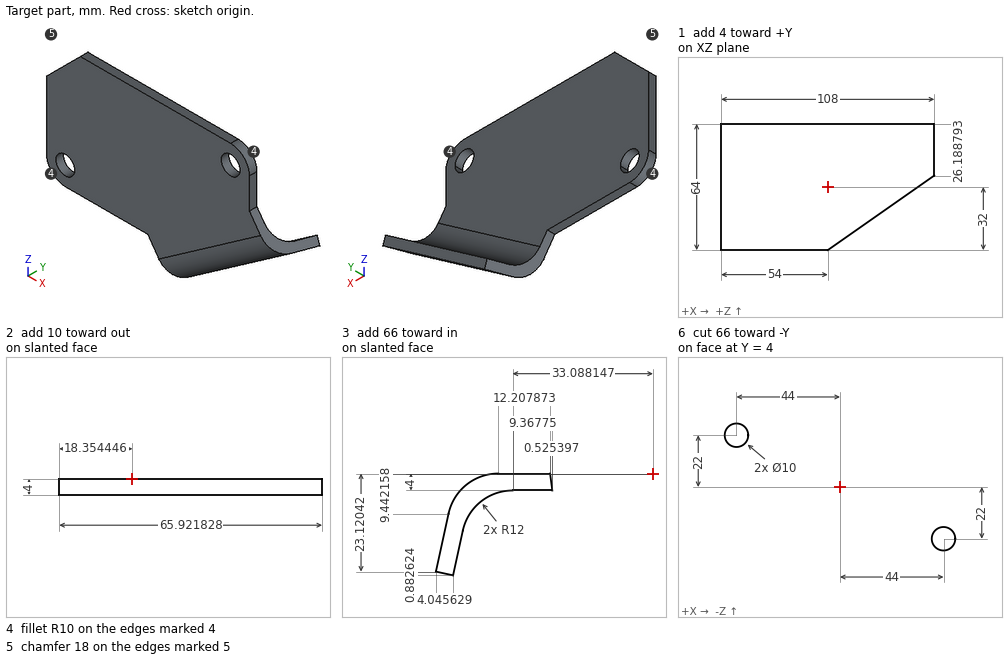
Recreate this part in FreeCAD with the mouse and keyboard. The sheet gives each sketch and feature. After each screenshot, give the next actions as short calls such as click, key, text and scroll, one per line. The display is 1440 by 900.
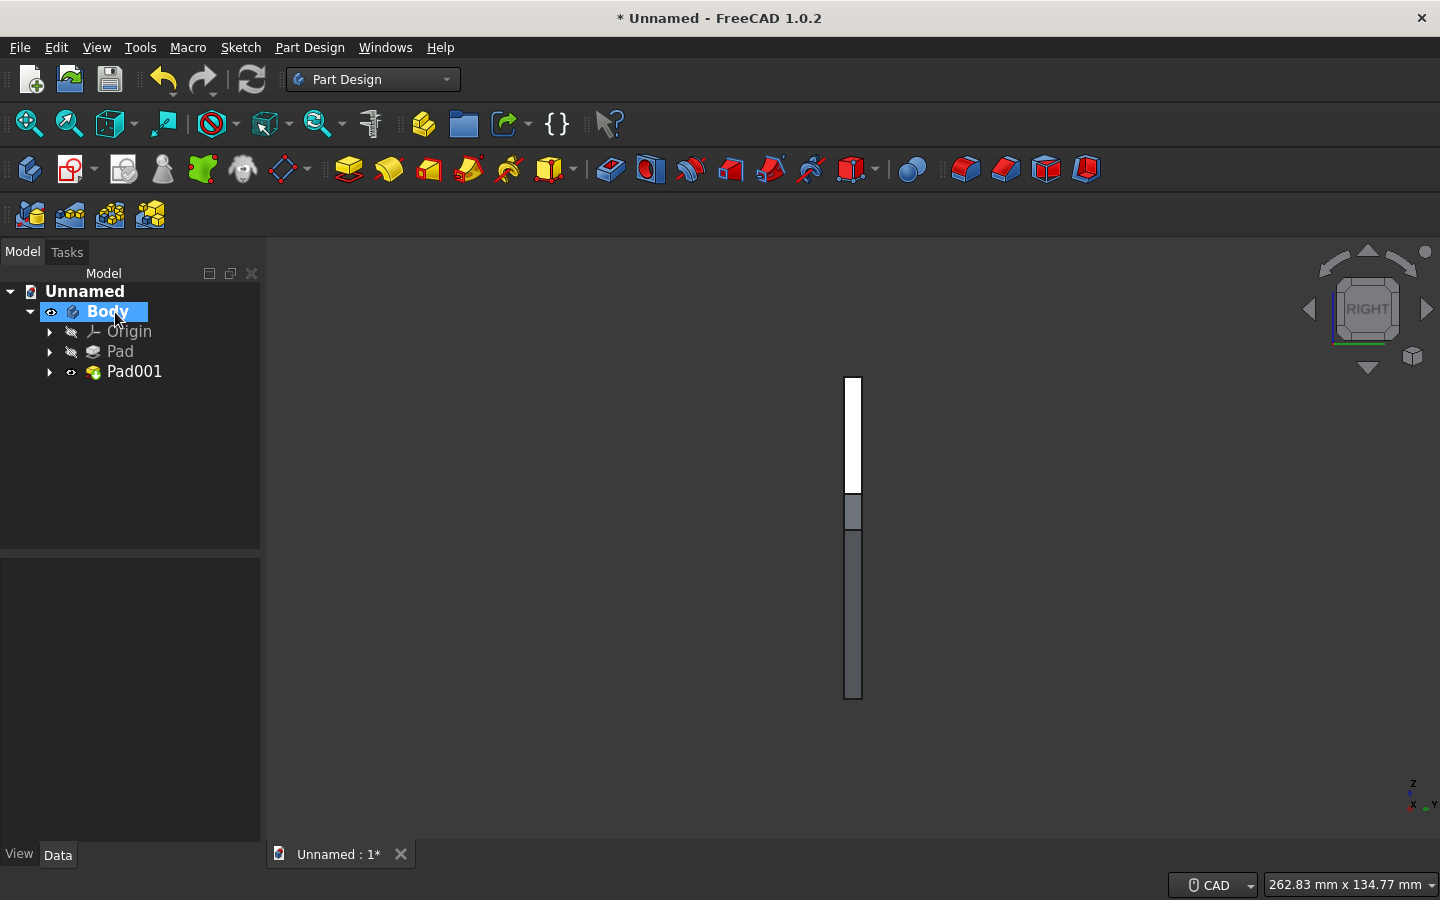
click(853, 516)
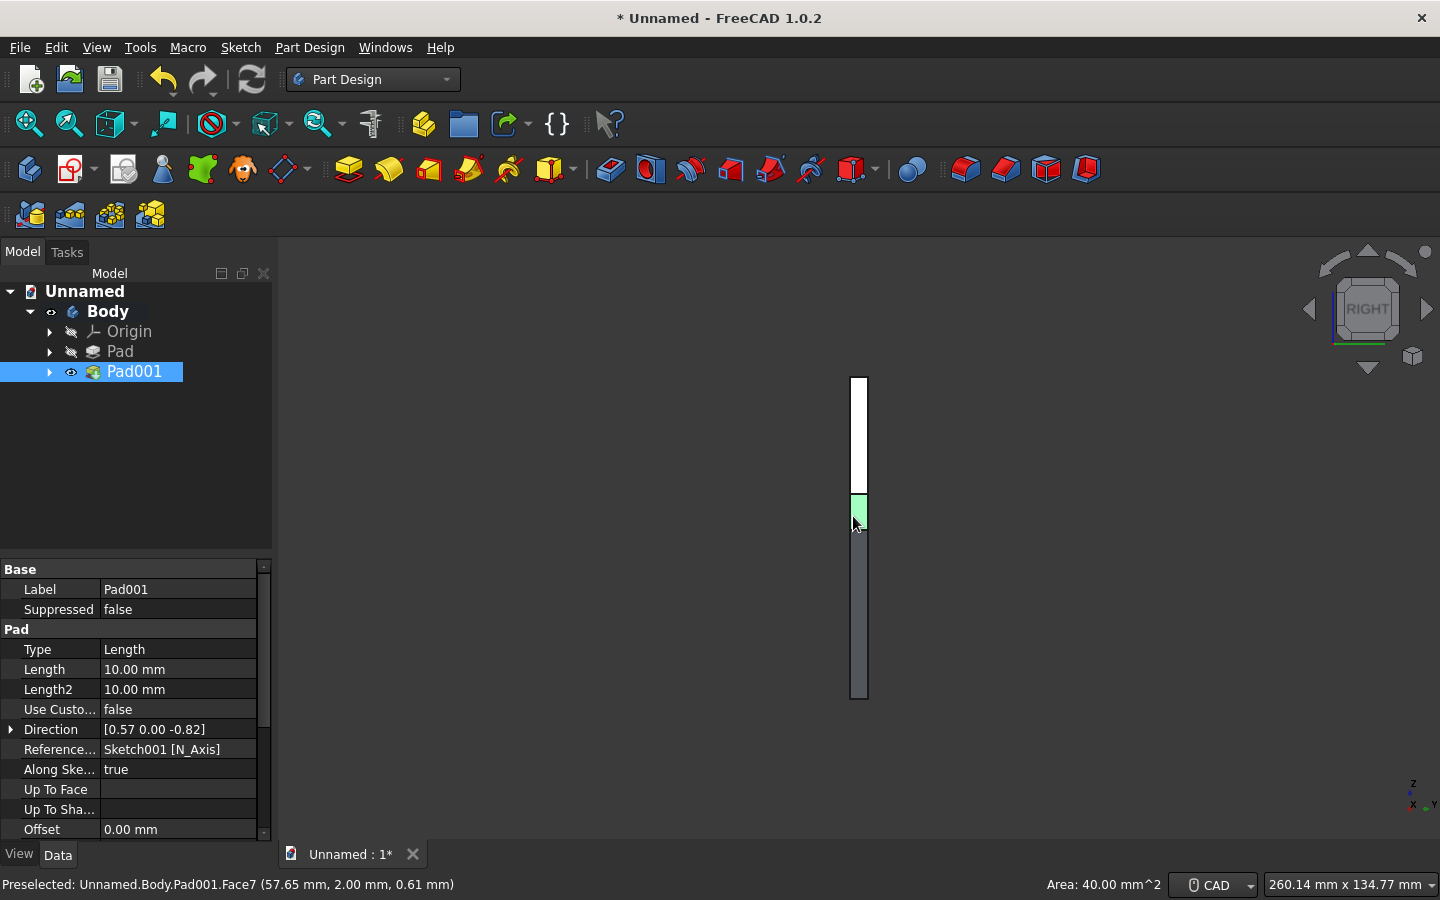
click(70, 170)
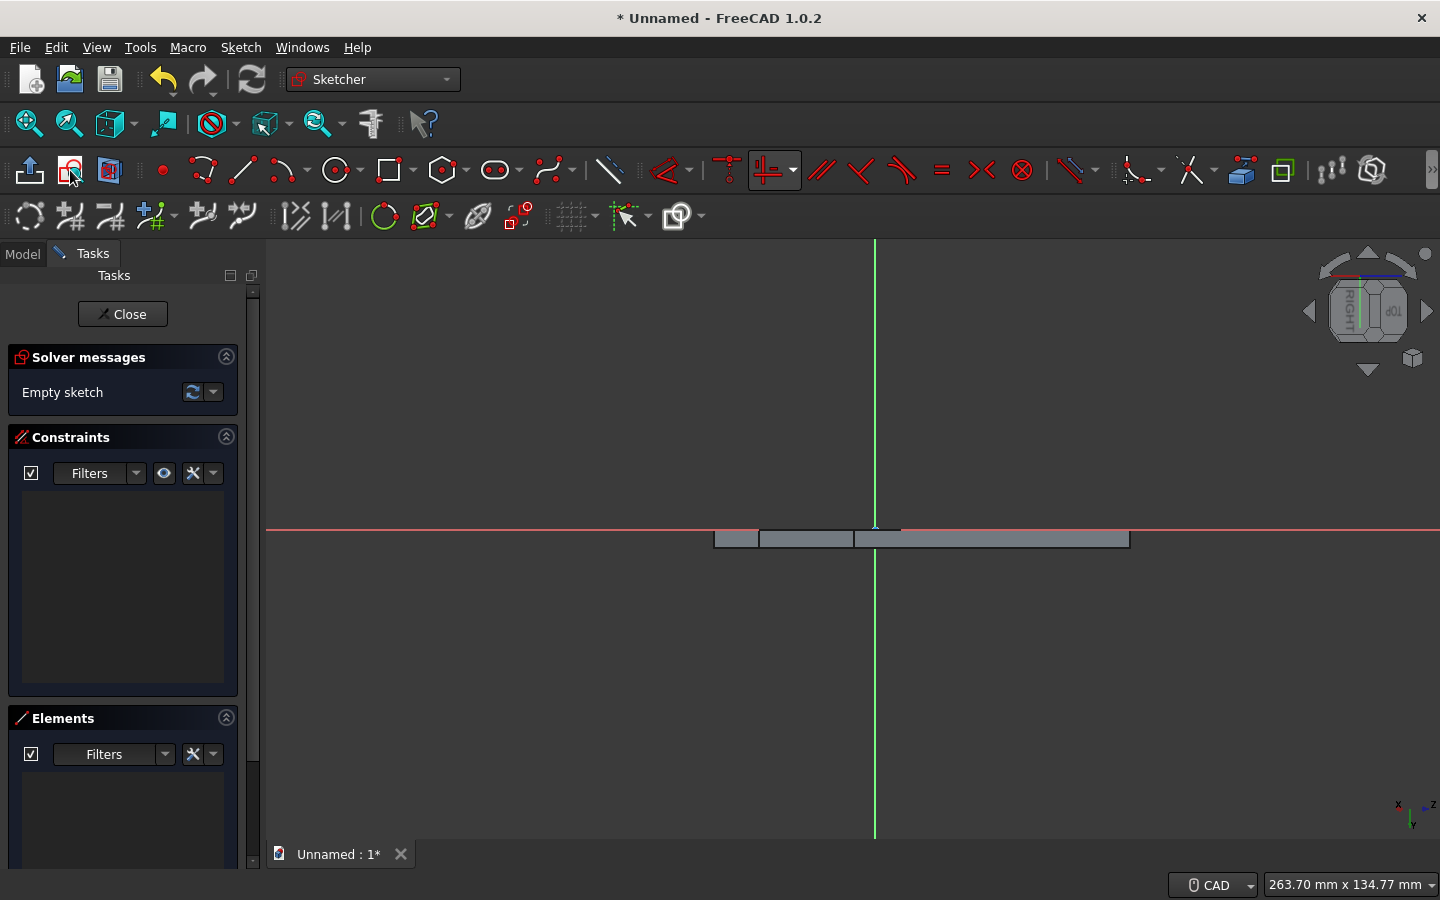
scroll(751, 603, up, 6)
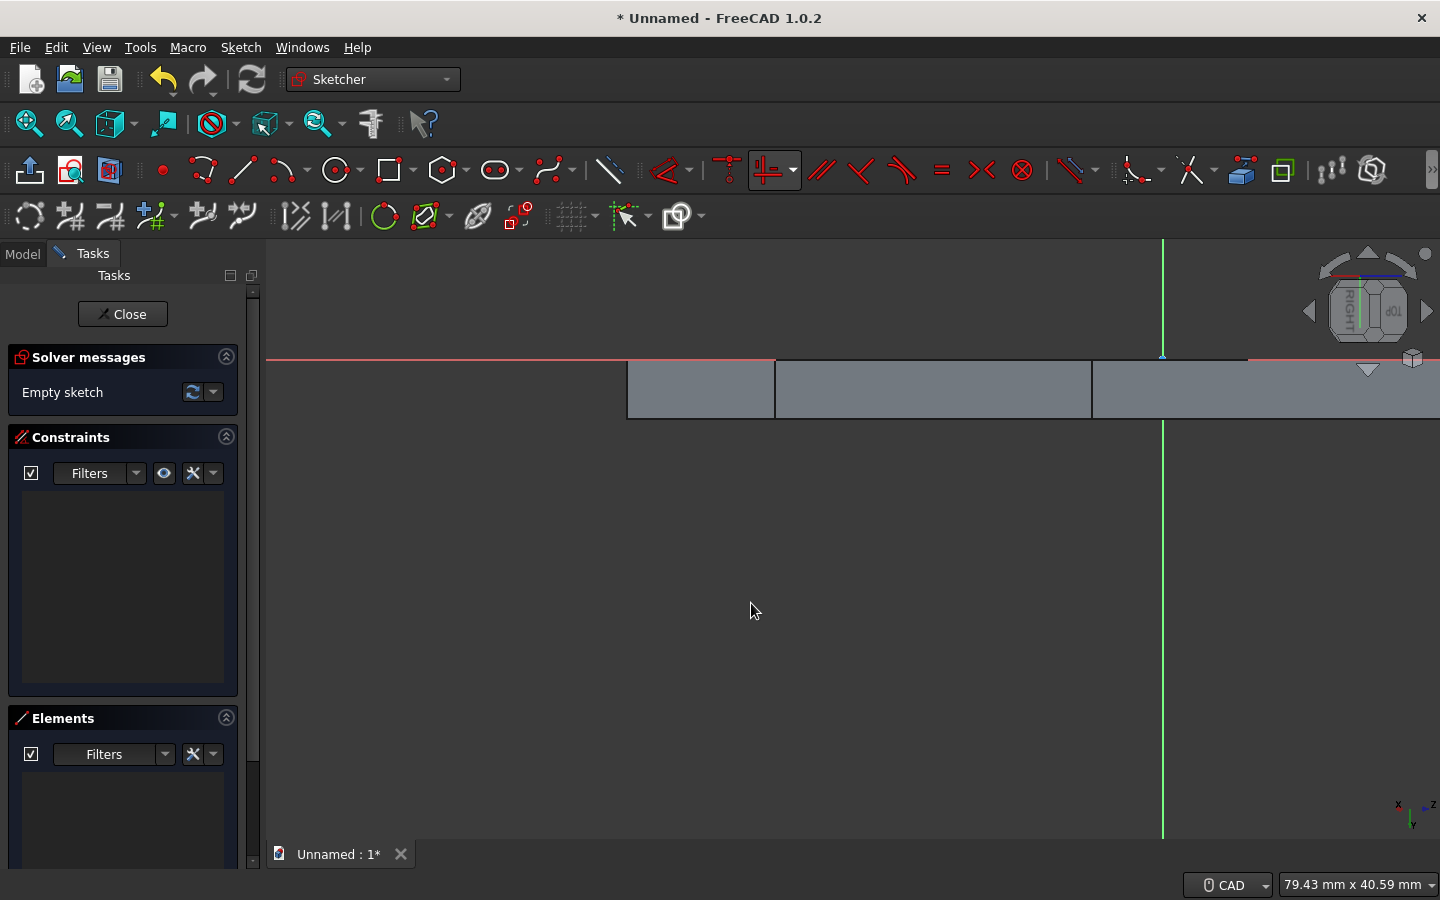
key(g)
key(m)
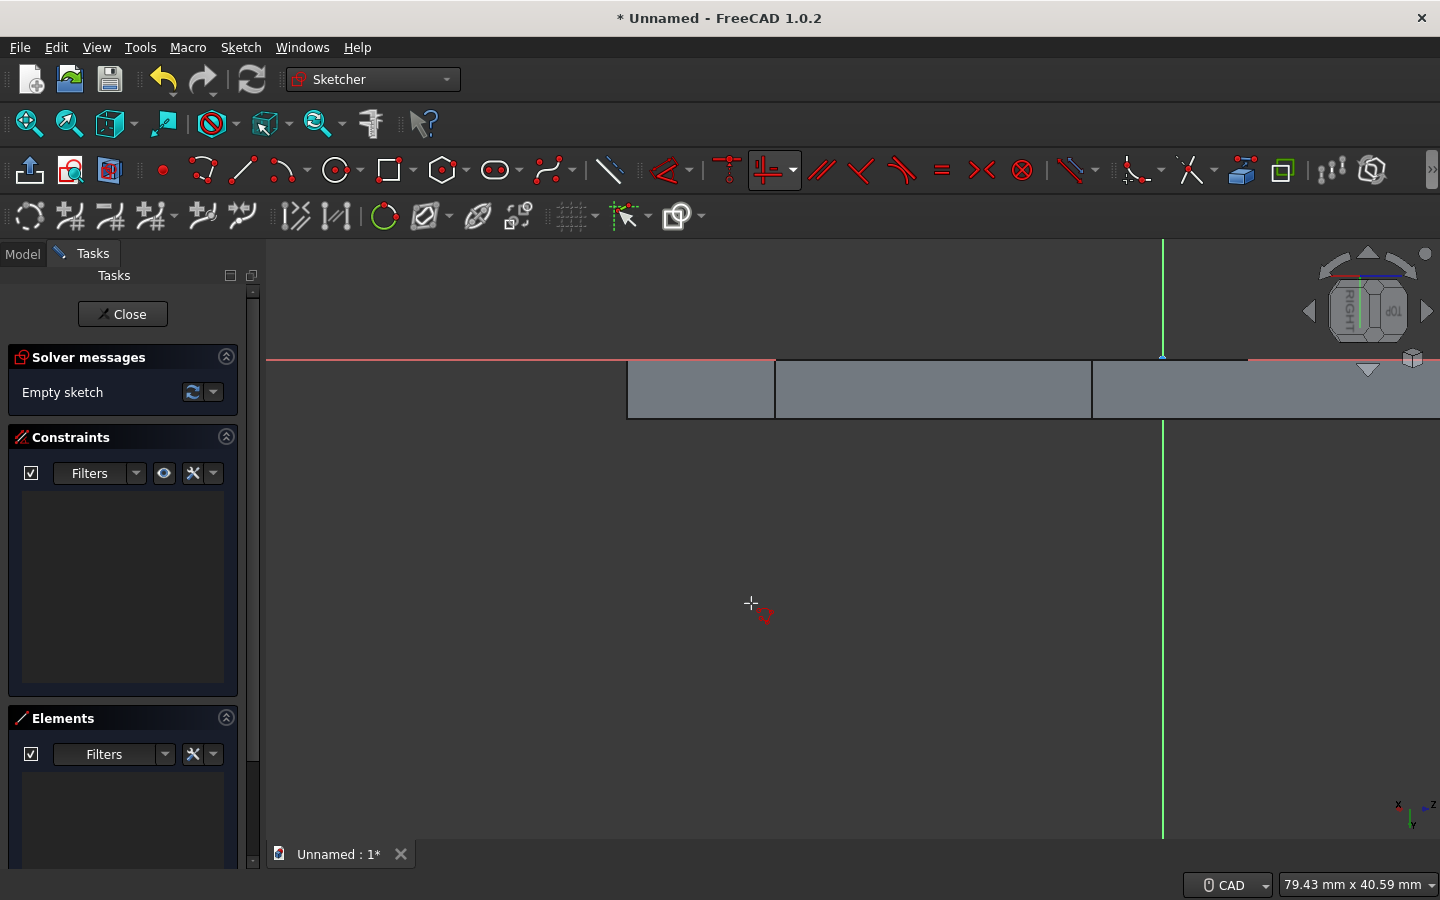
click(674, 419)
click(812, 419)
click(804, 360)
click(624, 369)
right_click(624, 369)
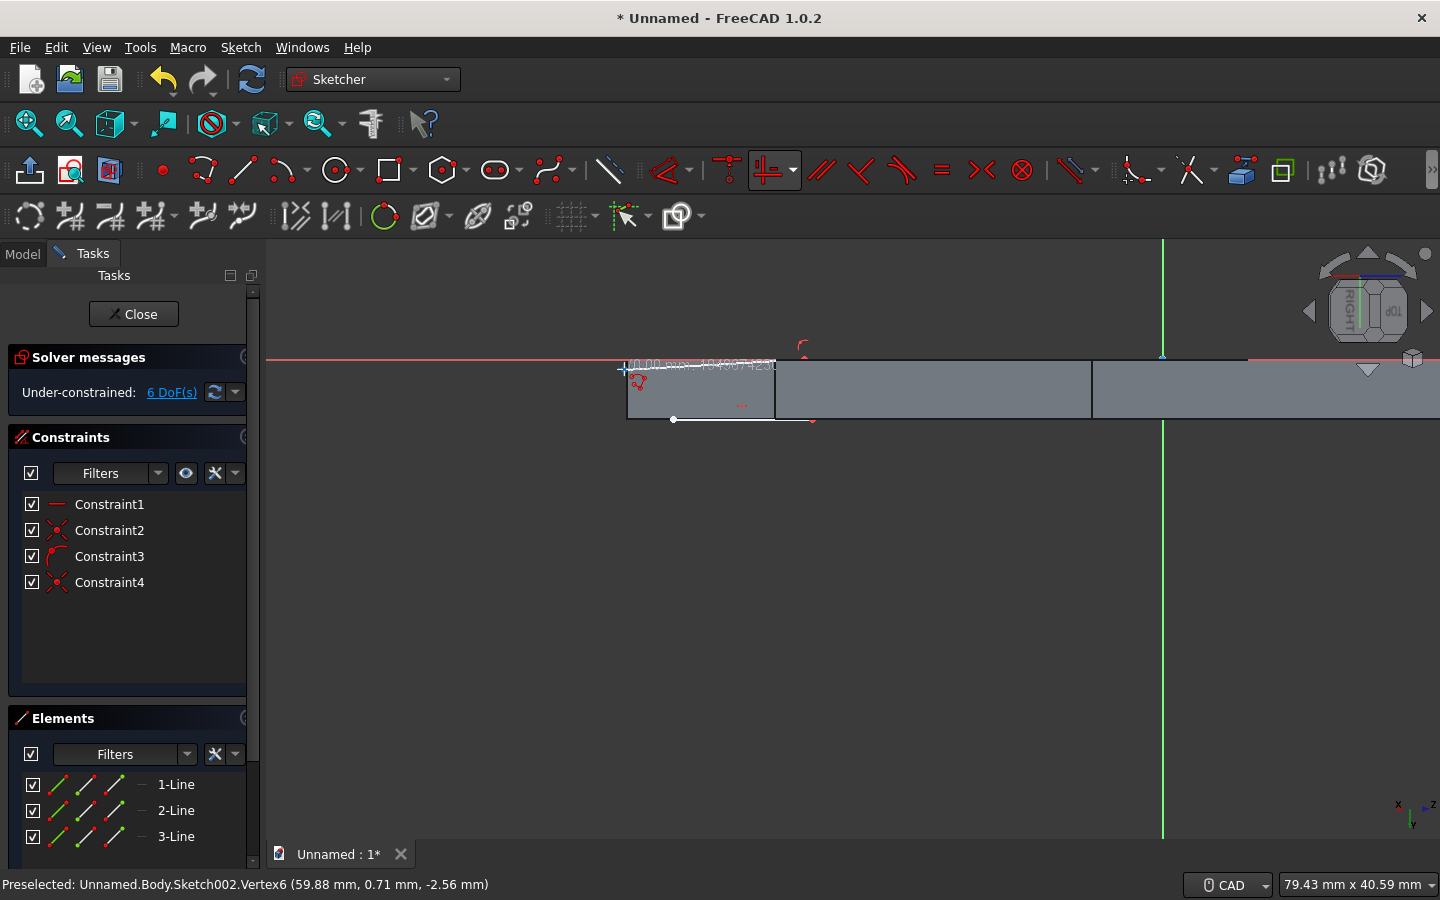
click(450, 499)
click(406, 701)
click(466, 714)
click(500, 558)
right_click(500, 558)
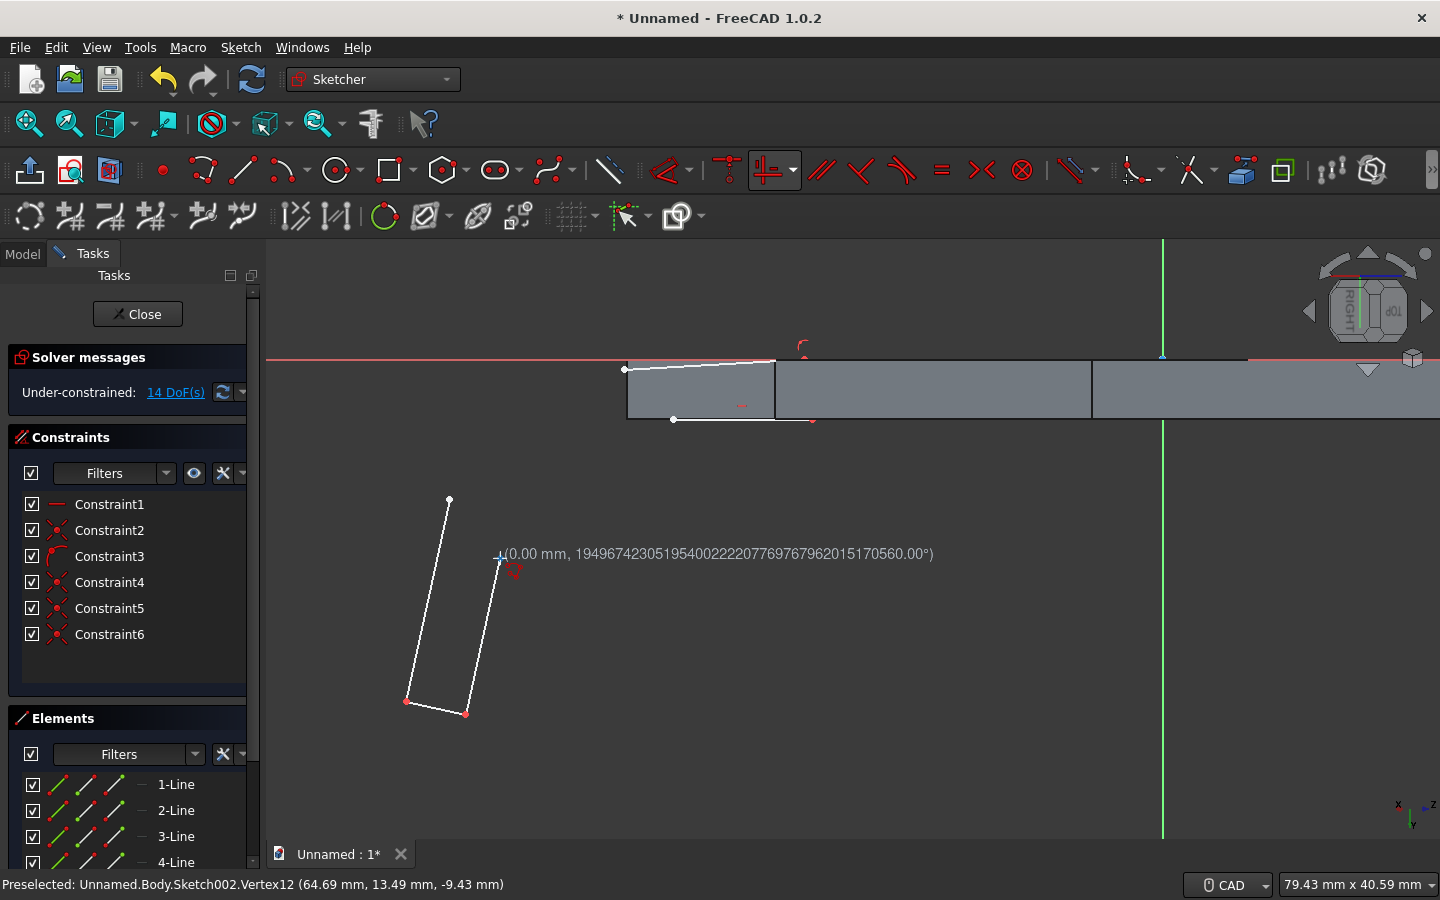
key(g)
key(3)
key(a)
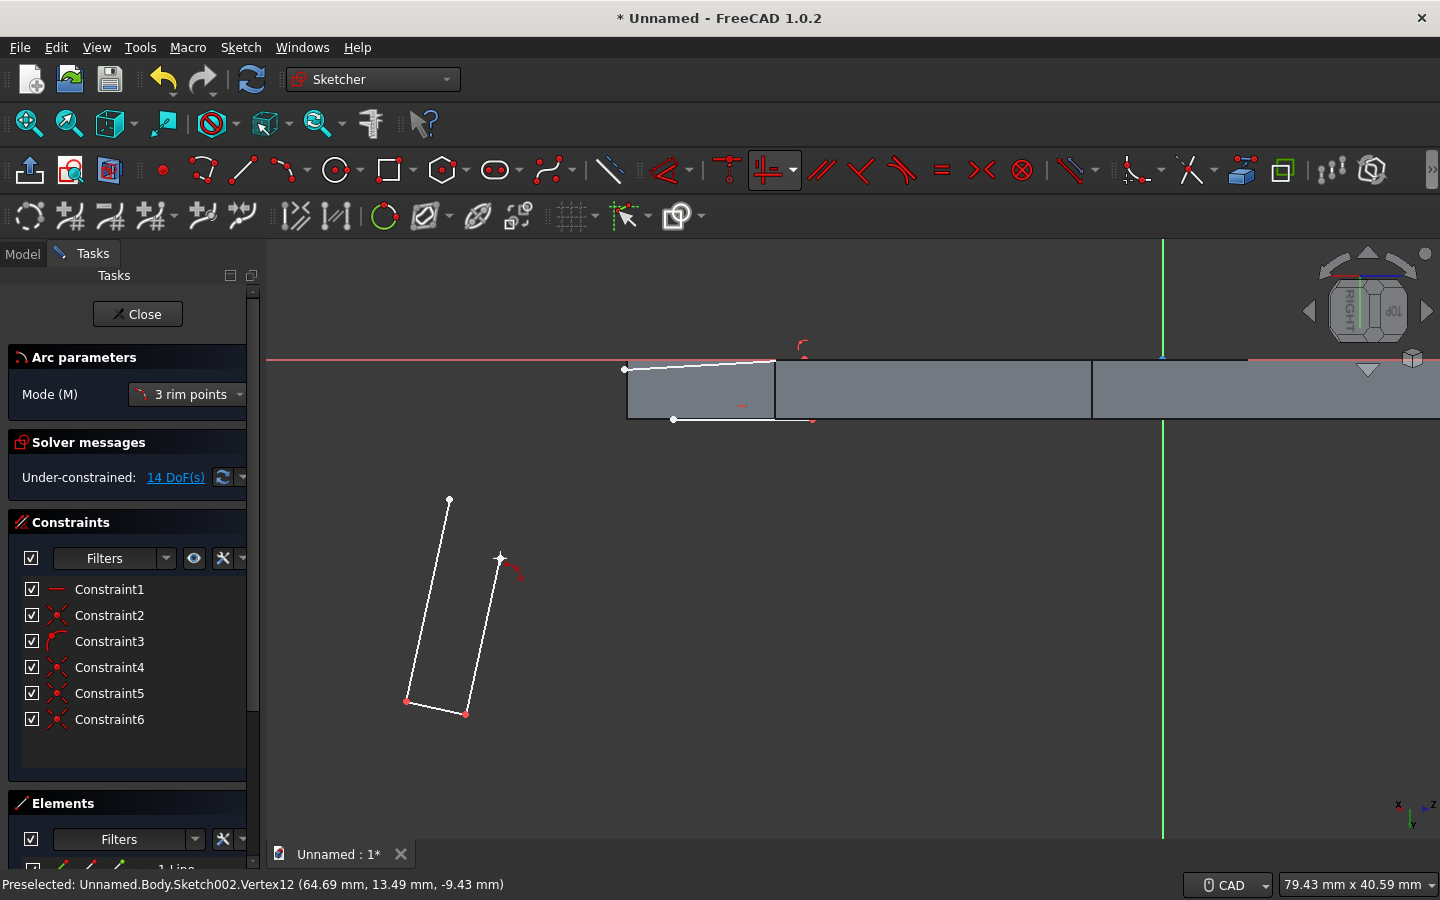
click(624, 370)
click(450, 500)
click(513, 399)